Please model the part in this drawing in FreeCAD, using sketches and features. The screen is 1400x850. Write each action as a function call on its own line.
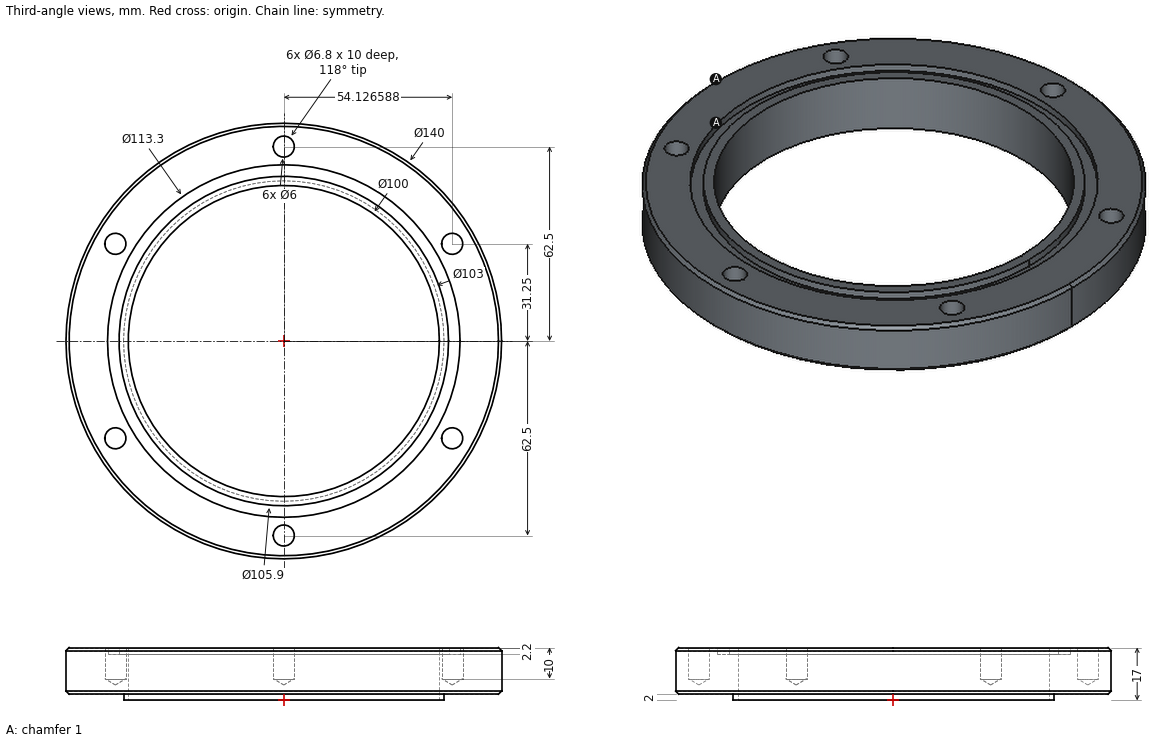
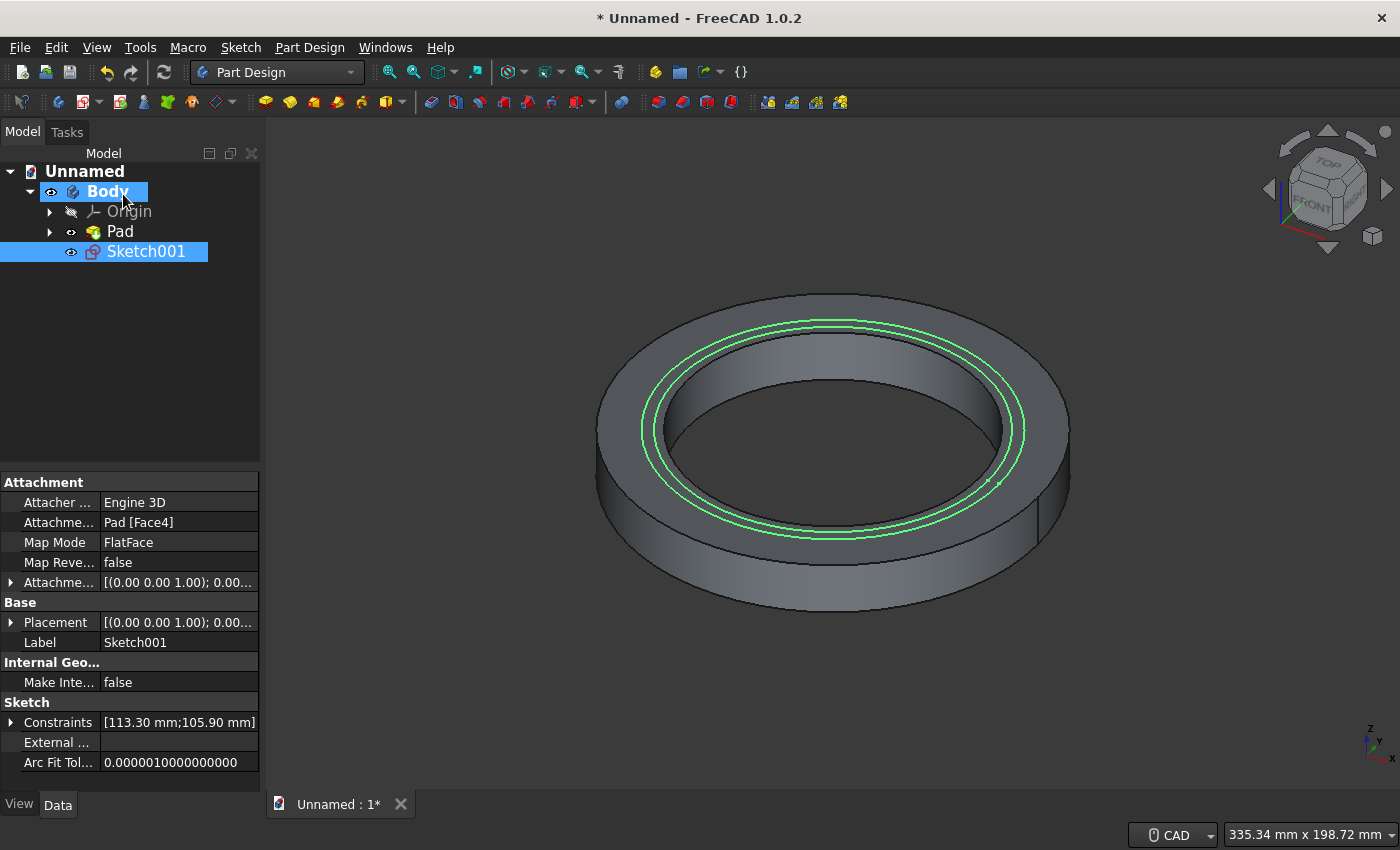
click(432, 102)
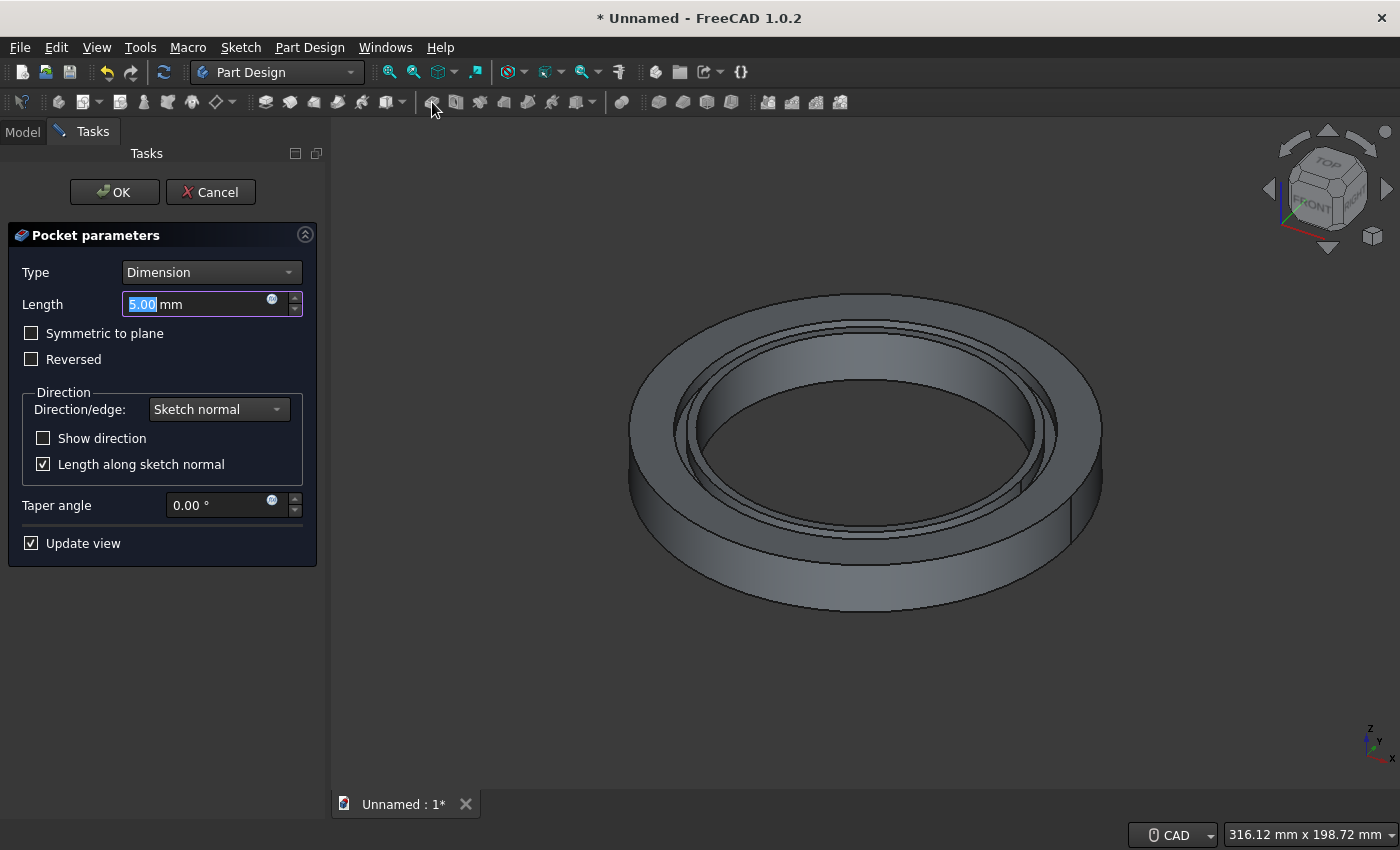
text(2.2)
key(Tab)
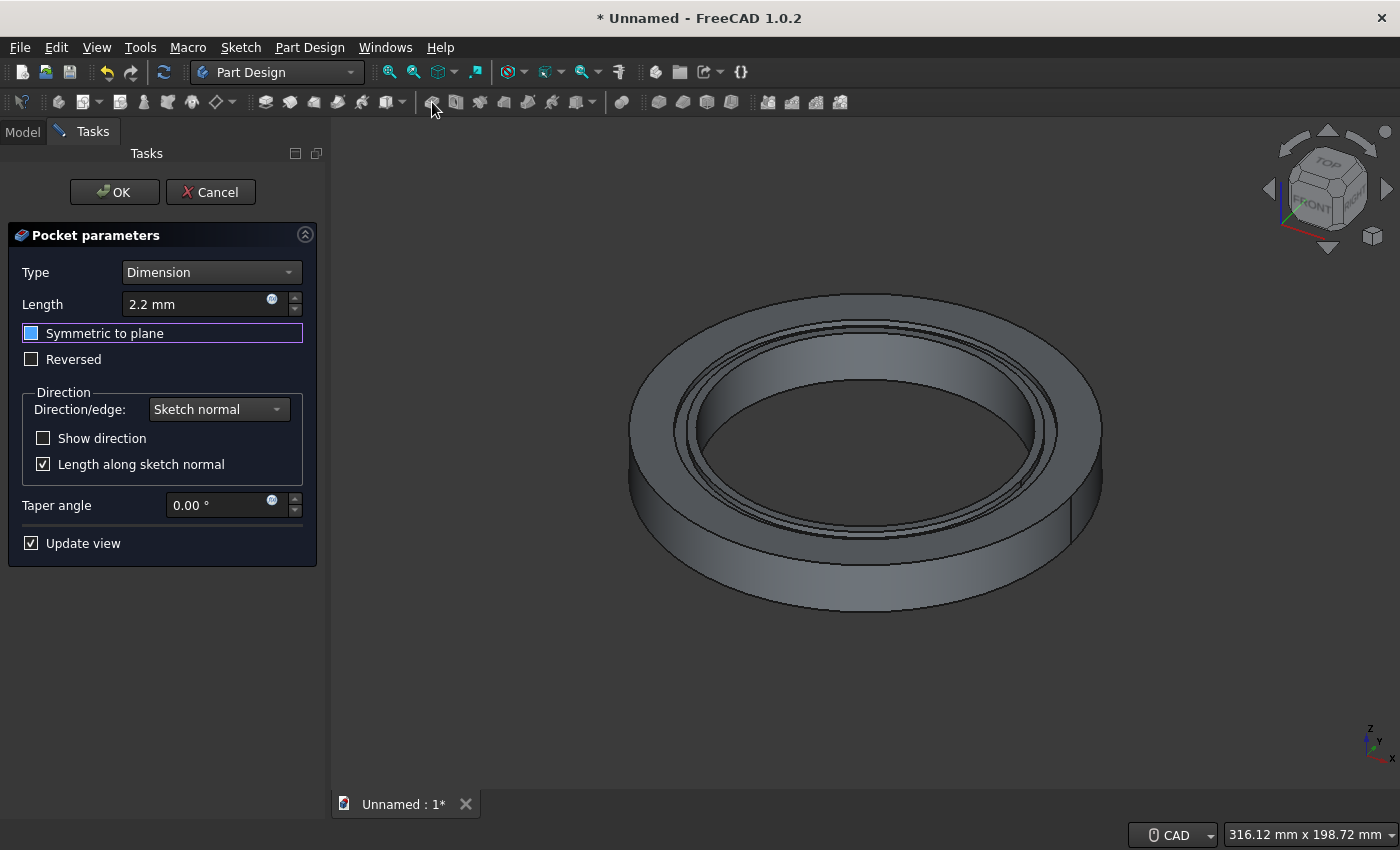
click(115, 192)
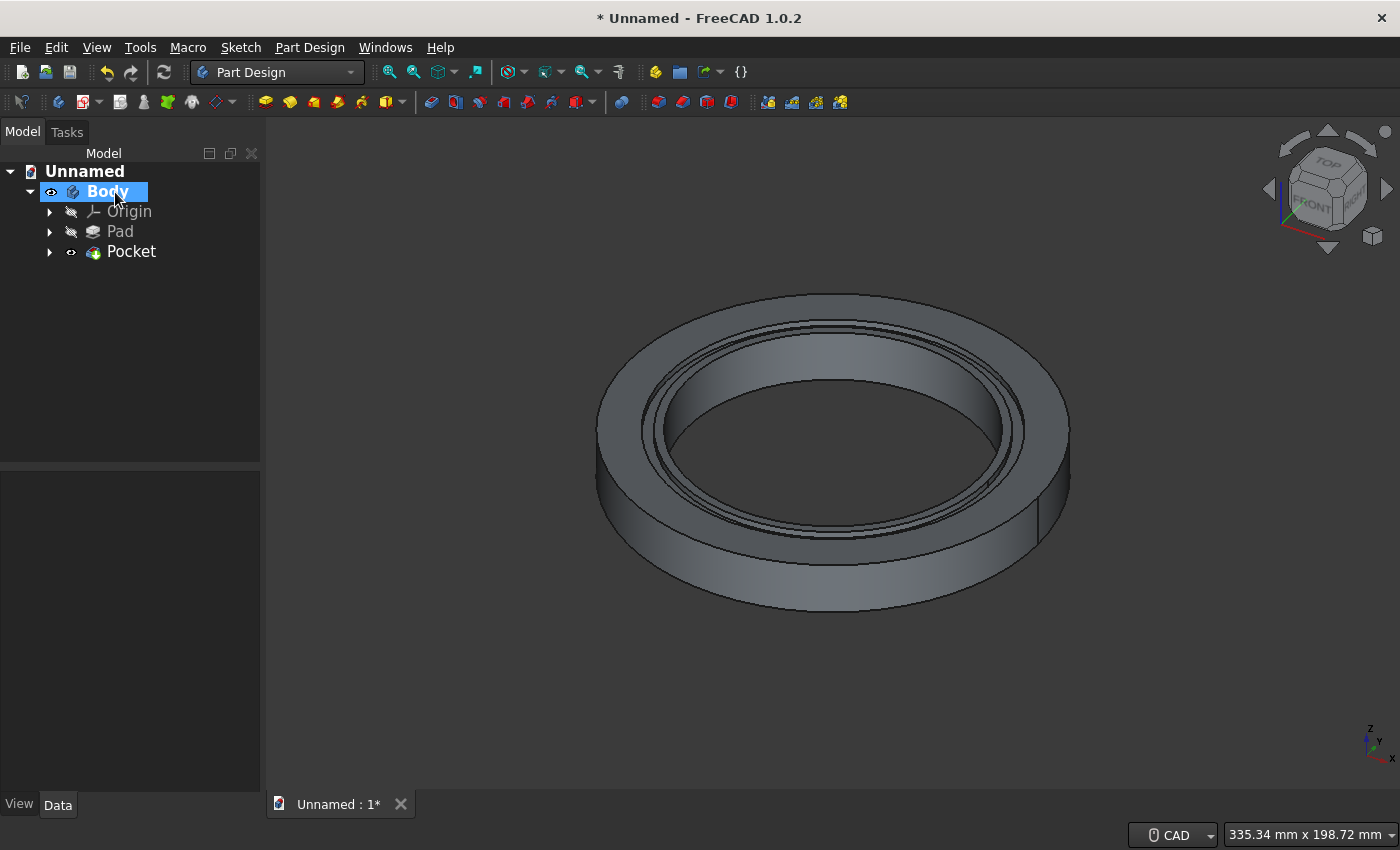
key(5)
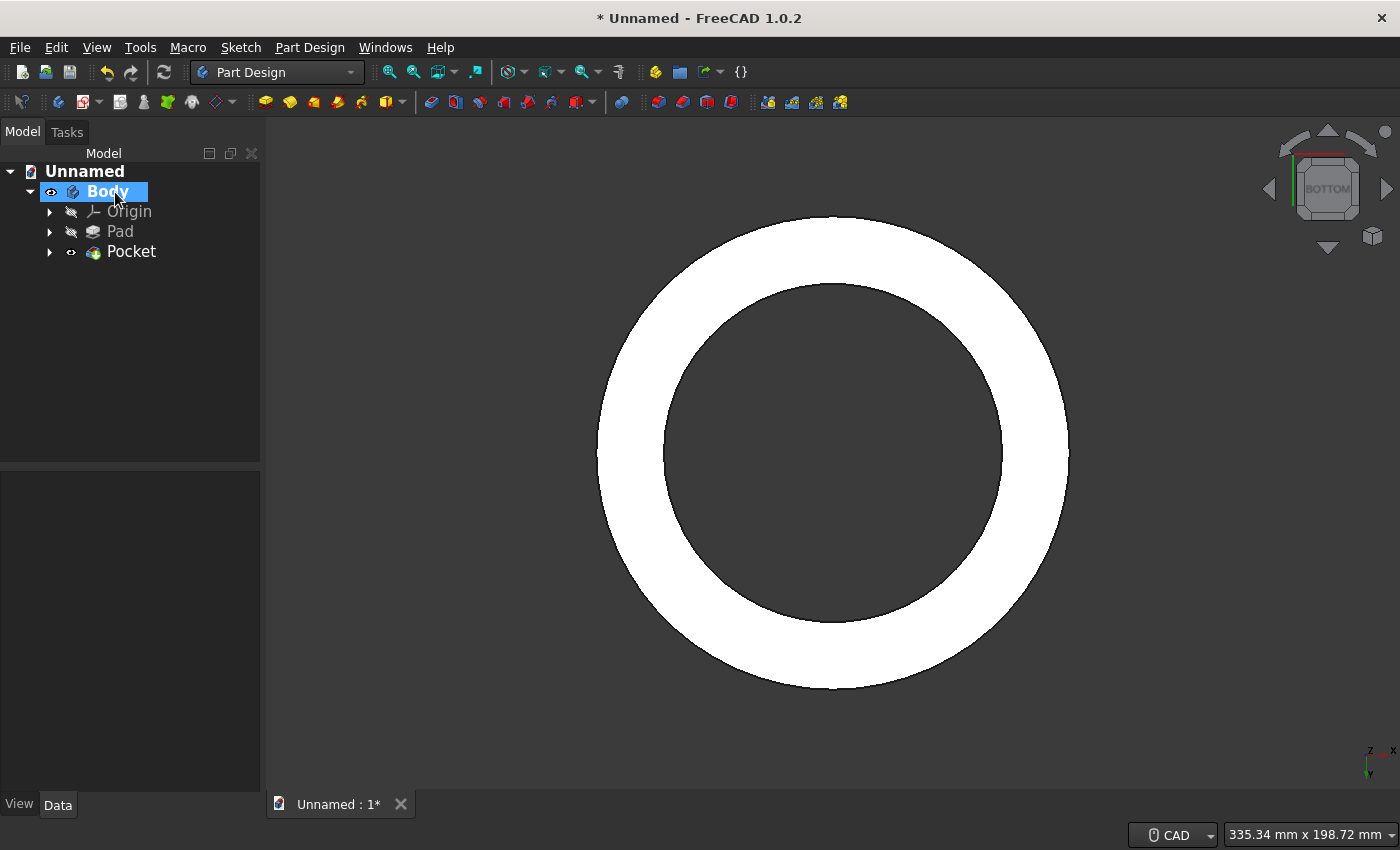
click(1036, 452)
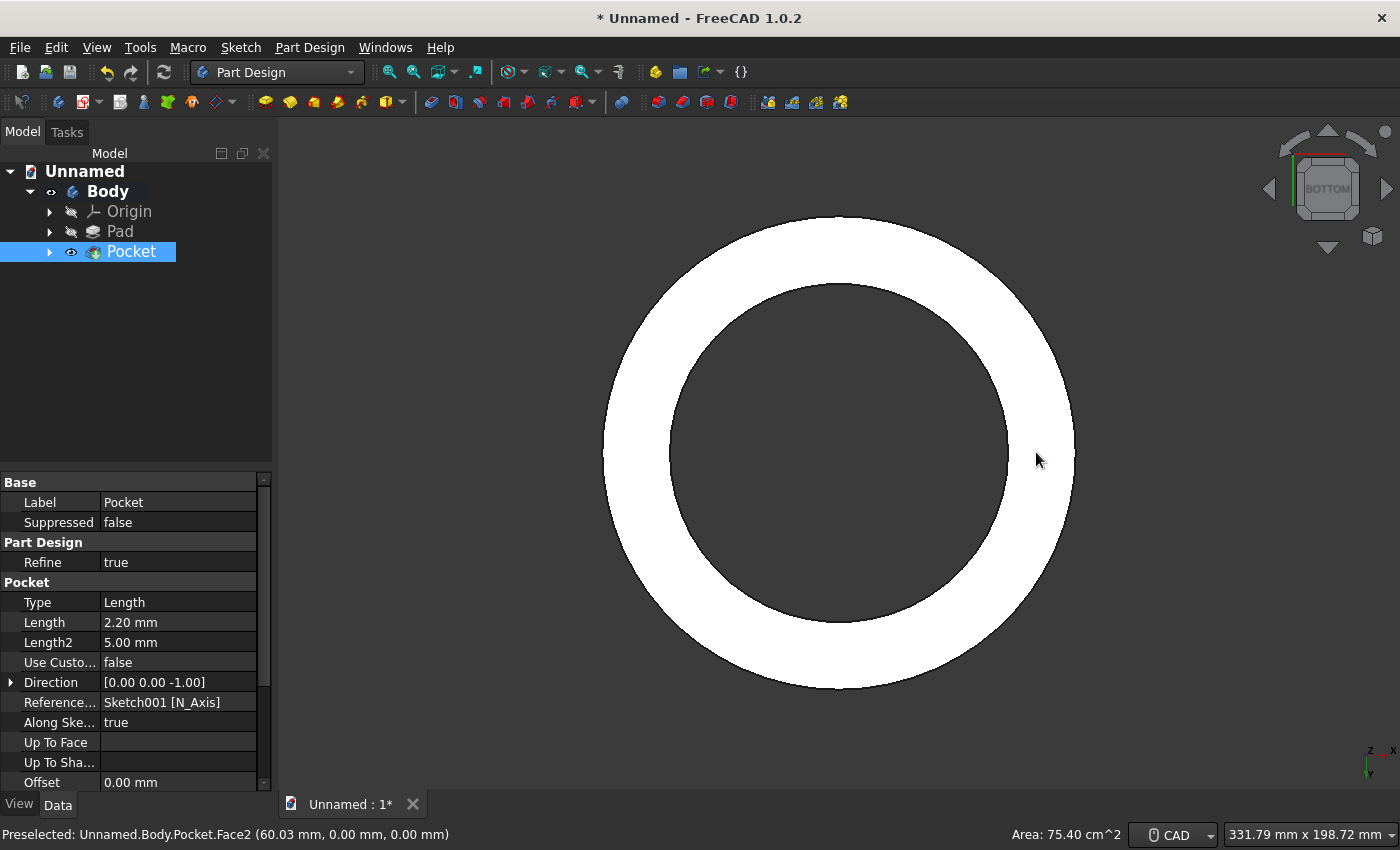
click(84, 102)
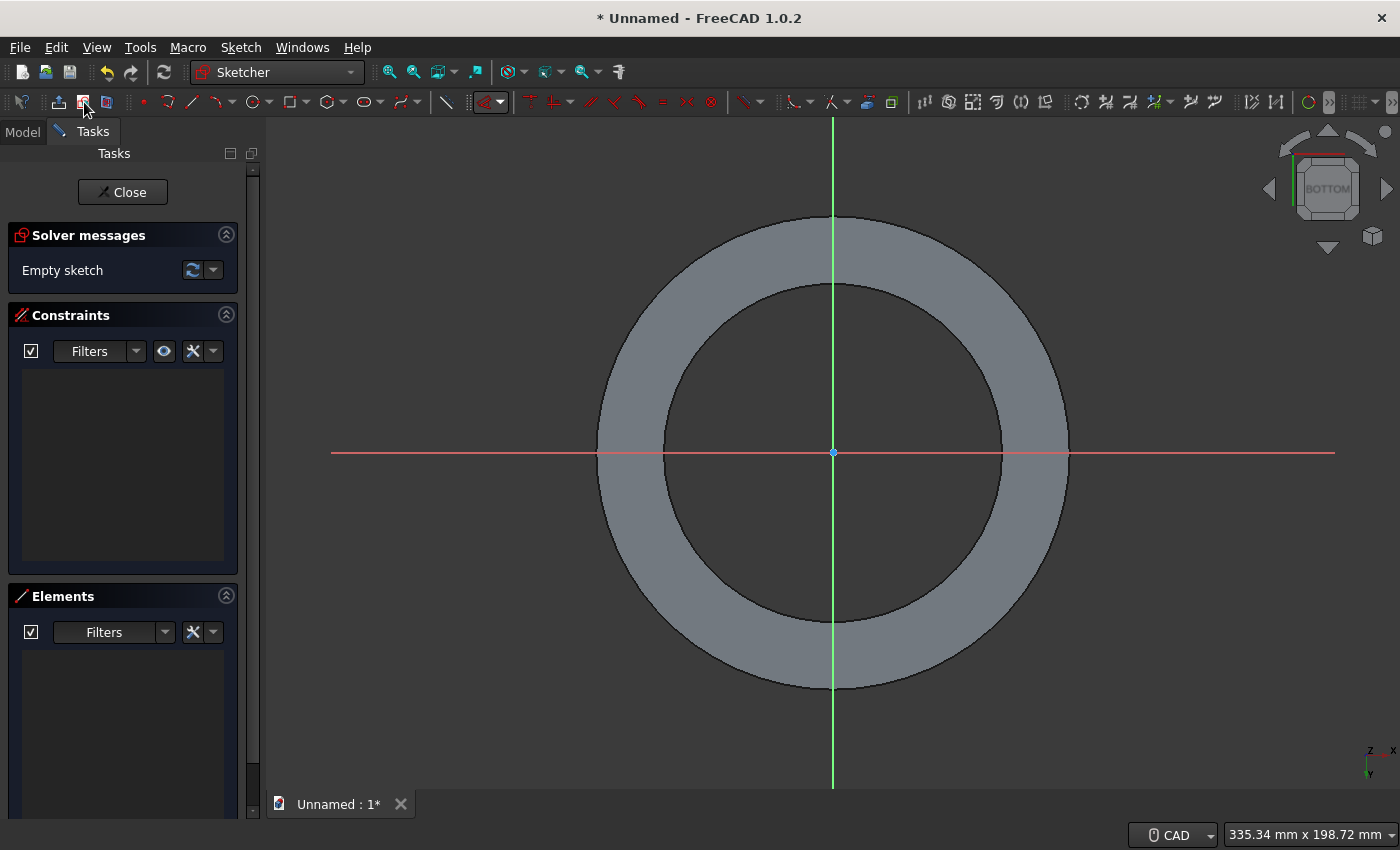
click(254, 102)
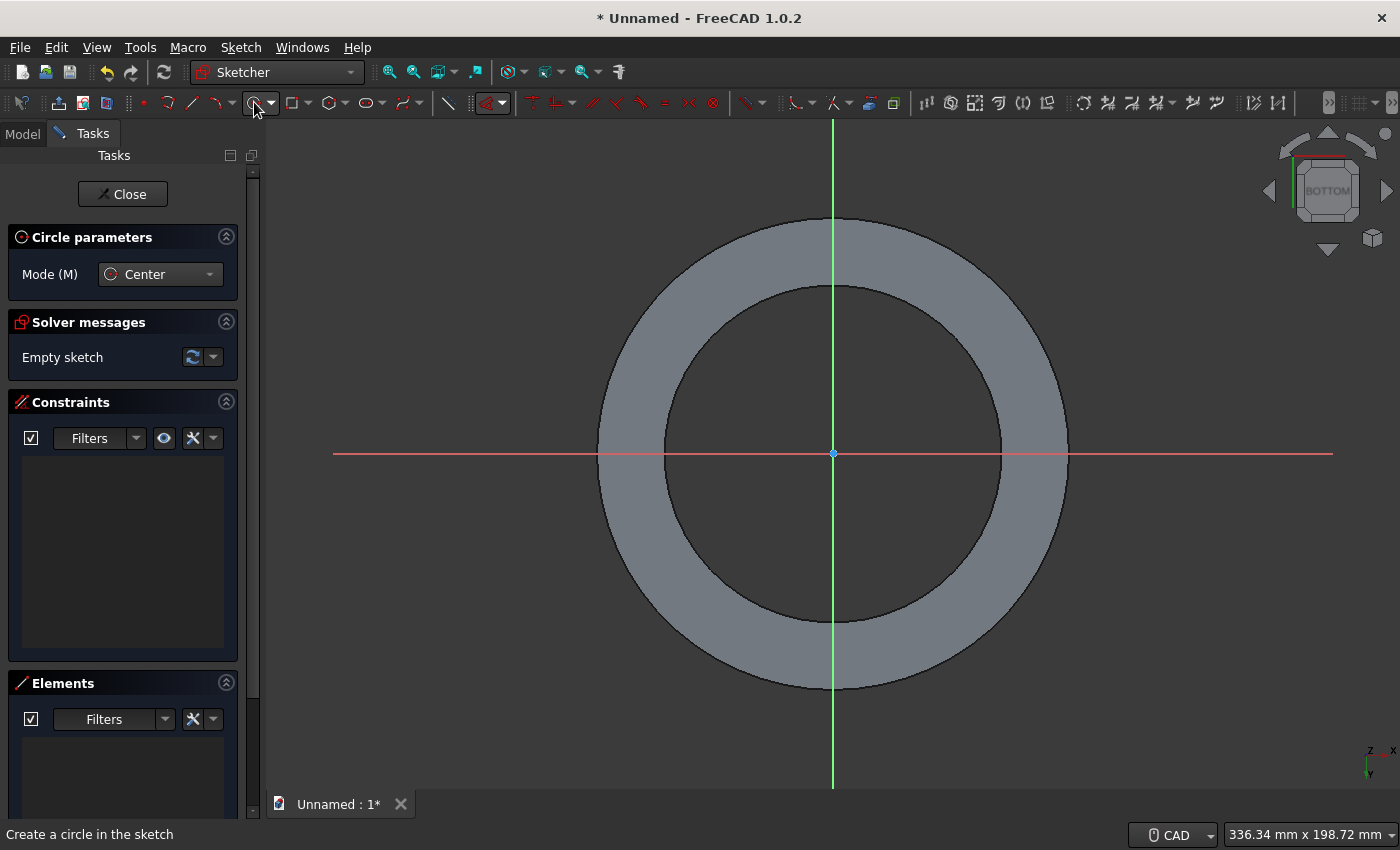
click(833, 454)
move(1000, 287)